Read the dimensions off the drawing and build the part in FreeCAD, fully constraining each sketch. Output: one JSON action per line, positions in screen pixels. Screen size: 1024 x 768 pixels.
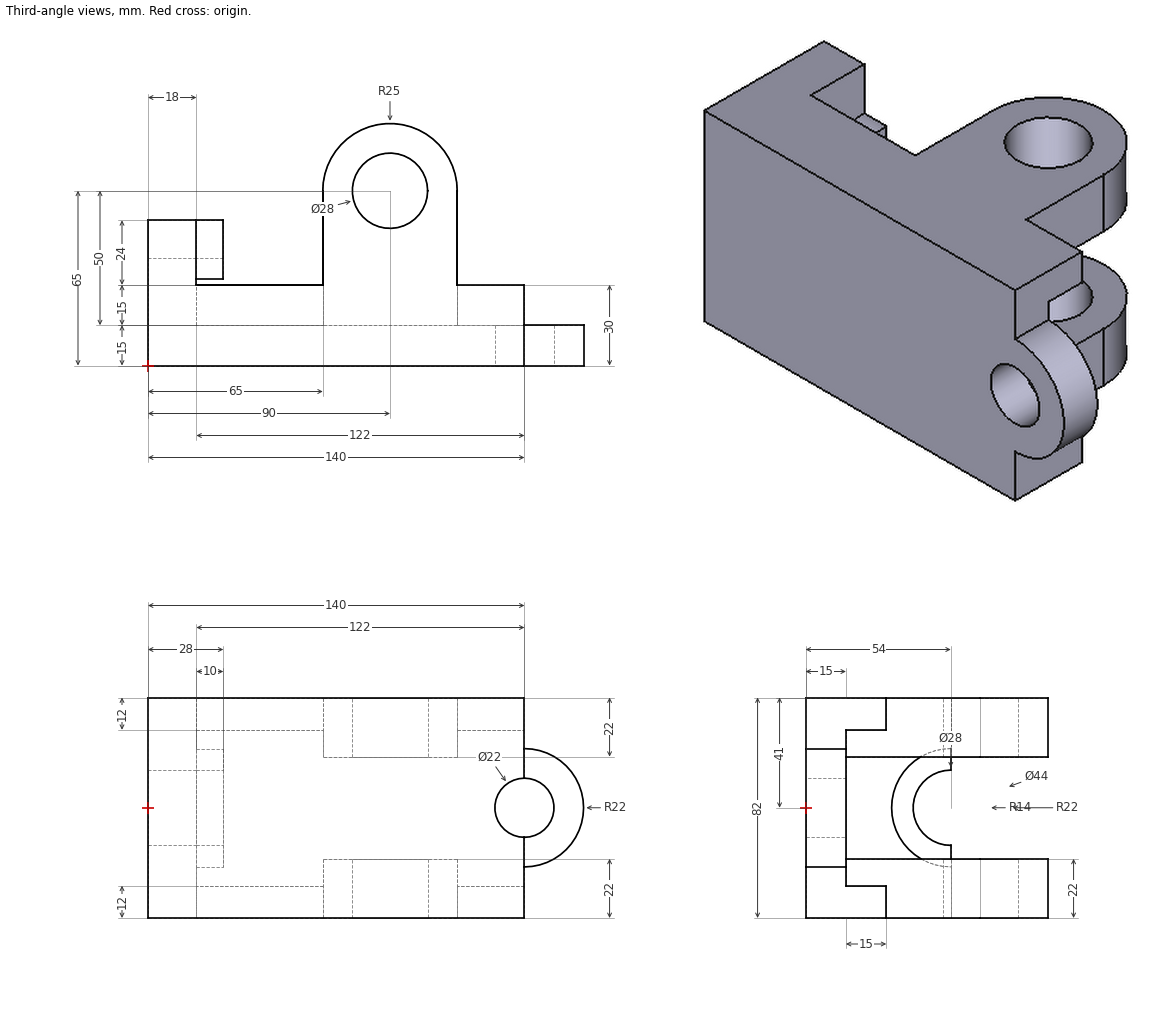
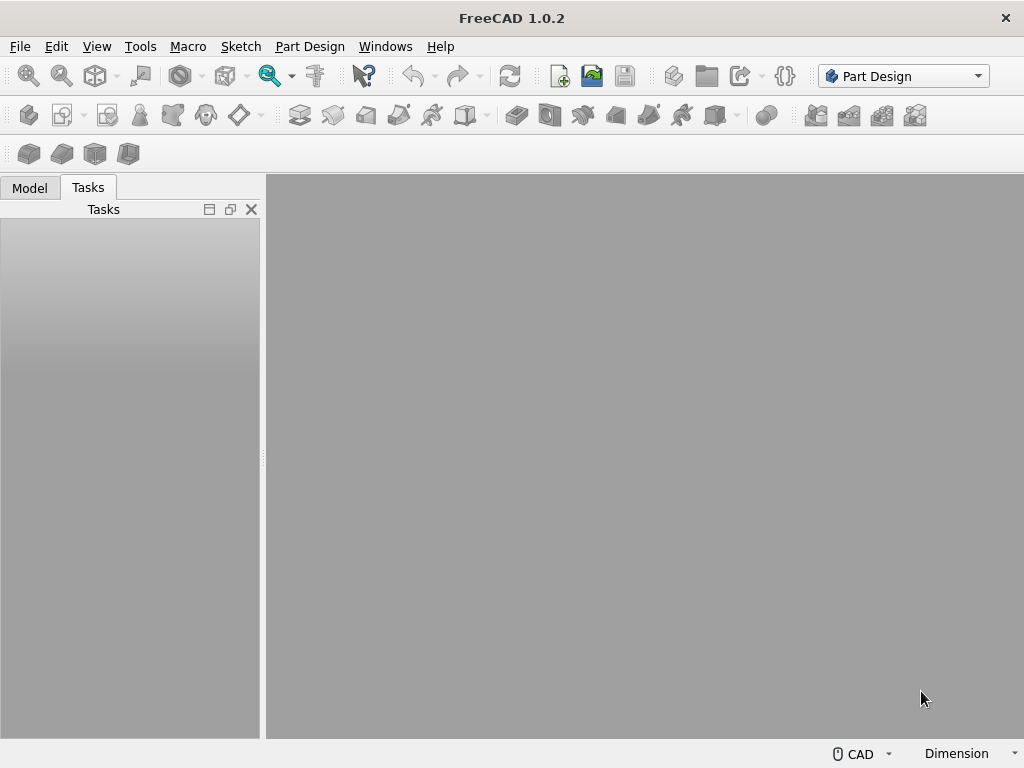
{"action": "key", "text": "ctrl+n"}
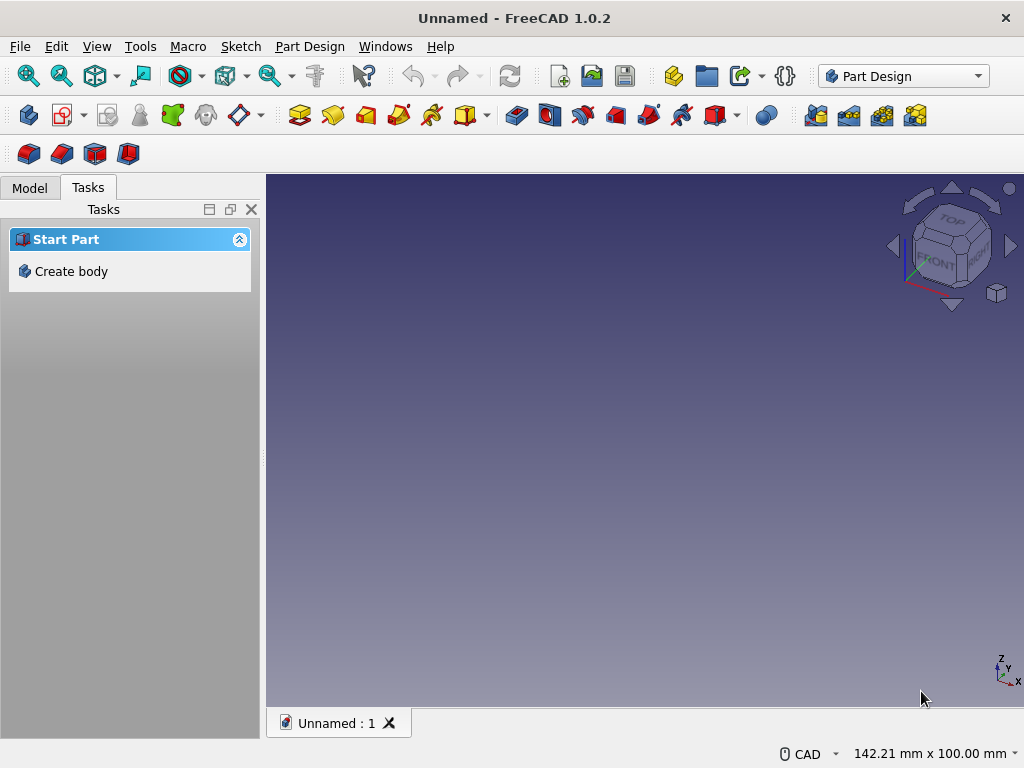
{"action": "left_click", "coordinate": [62, 116]}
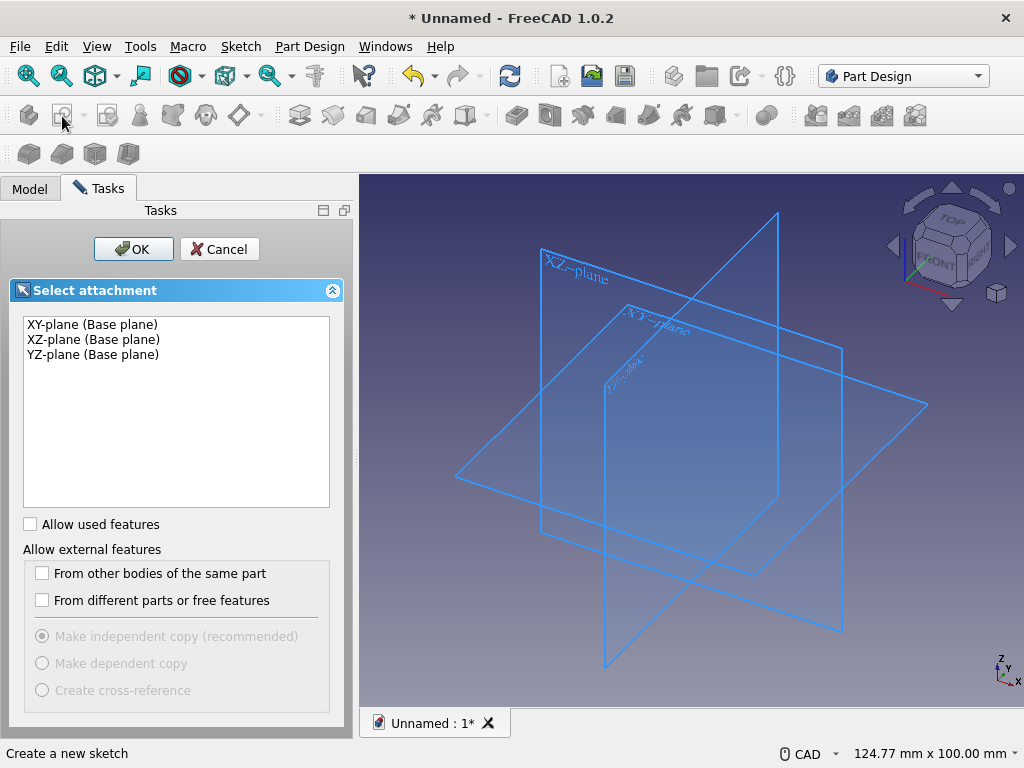
{"action": "left_click", "coordinate": [84, 324]}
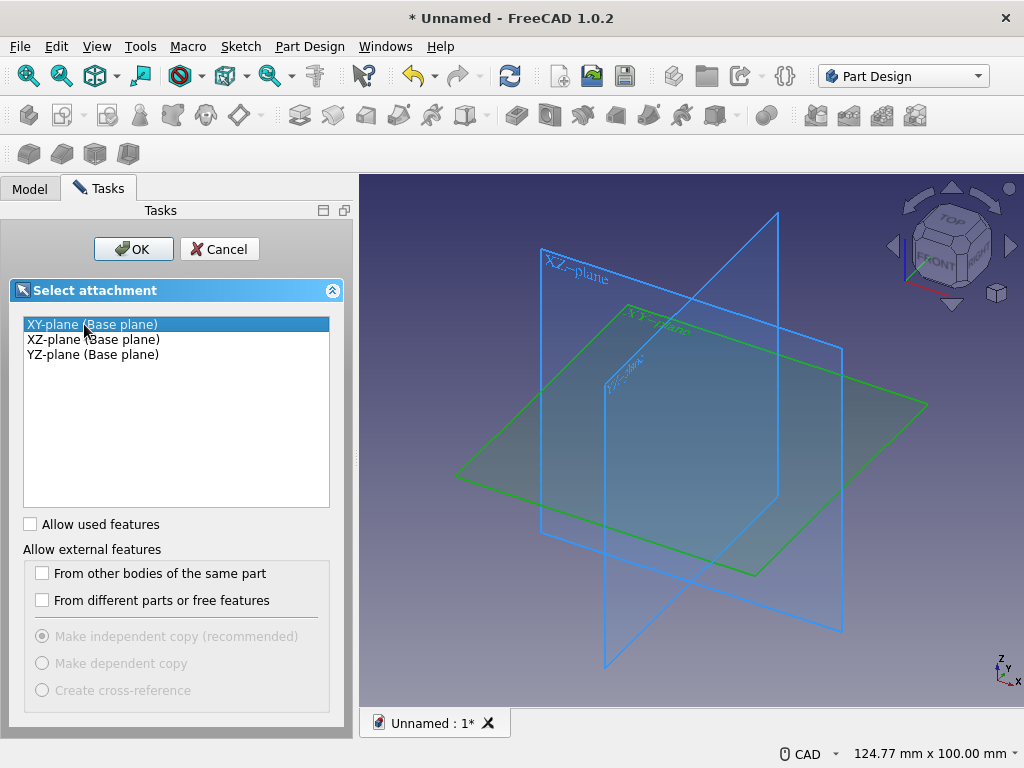
{"action": "left_click", "coordinate": [134, 249]}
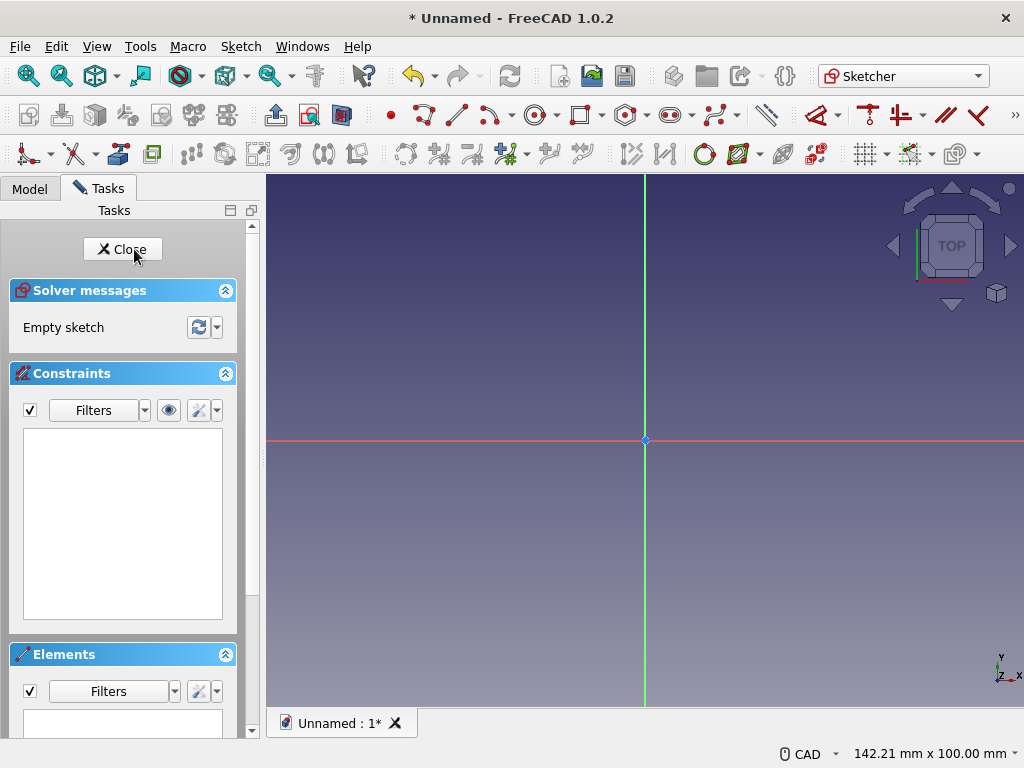
{"action": "scroll", "coordinate": [294, 558], "scroll_direction": "down", "scroll_amount": 4}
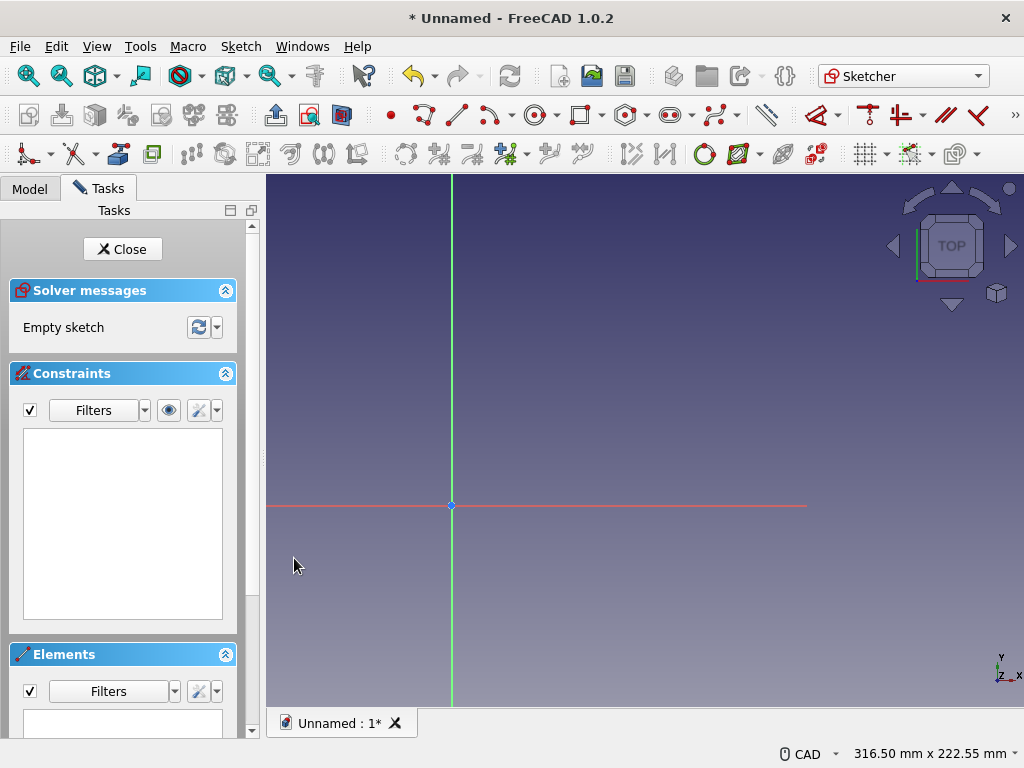
{"action": "left_click", "coordinate": [424, 116]}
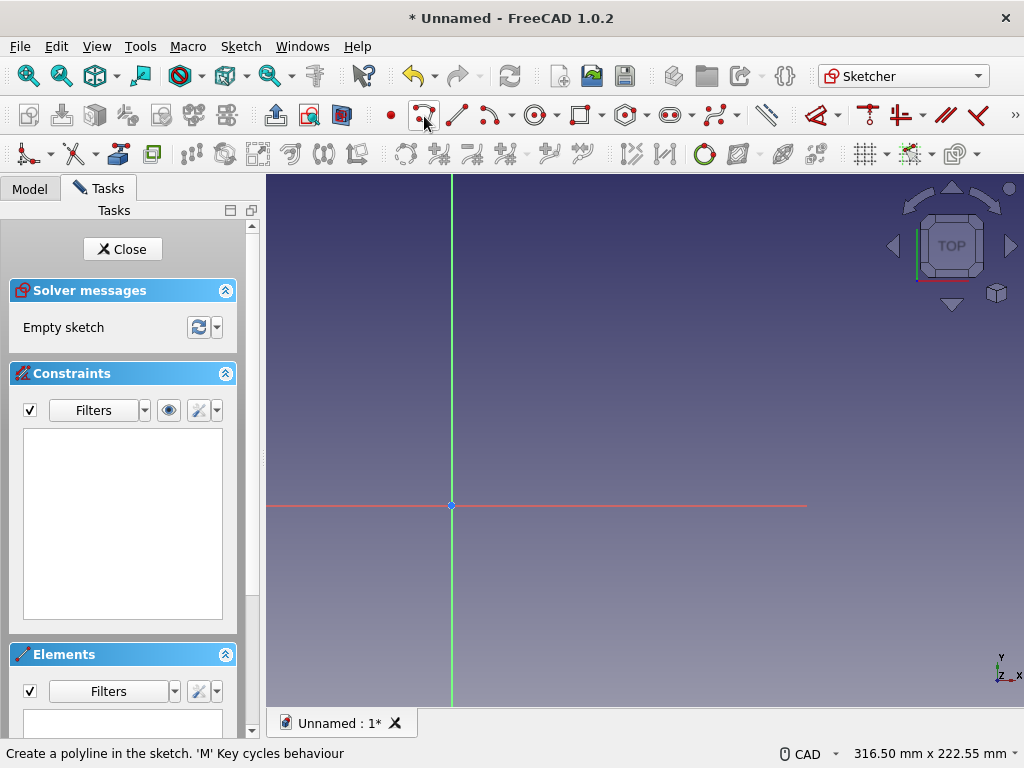
{"action": "left_click", "coordinate": [452, 506]}
{"action": "left_click", "coordinate": [787, 497]}
{"action": "left_click", "coordinate": [787, 434]}
{"action": "left_click", "coordinate": [495, 434]}
{"action": "left_click", "coordinate": [495, 376]}
{"action": "left_click", "coordinate": [461, 376]}
{"action": "left_click", "coordinate": [452, 506]}
{"action": "key", "text": "Escape"}
{"action": "key", "text": "Escape"}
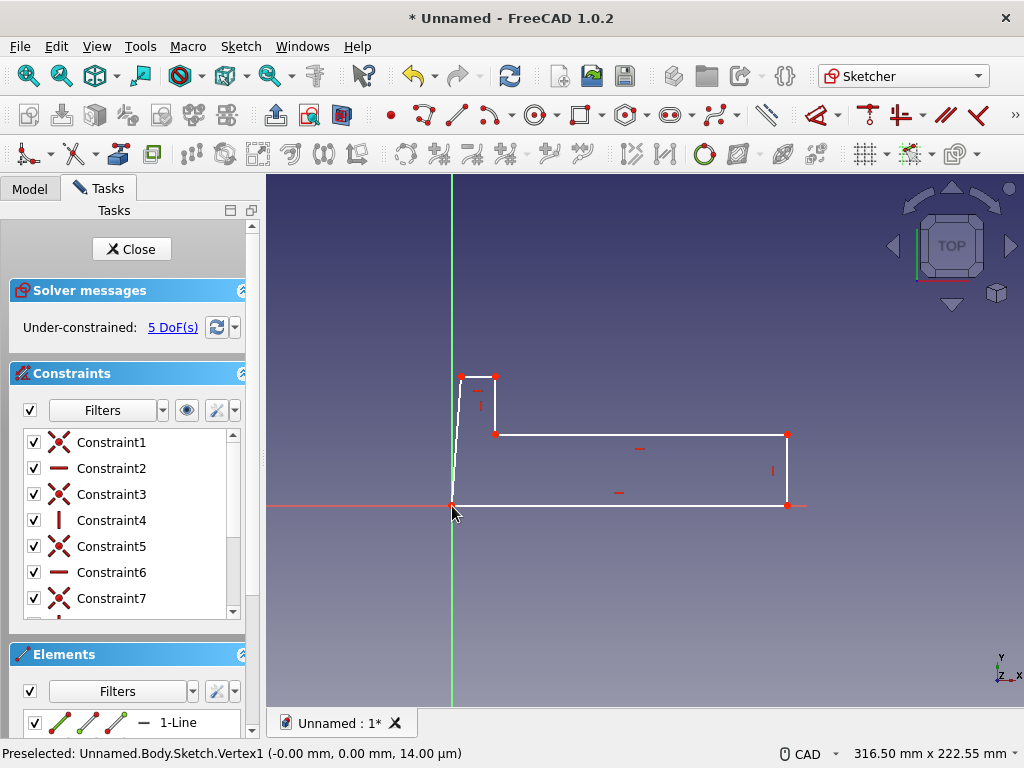
{"action": "left_click", "coordinate": [455, 467]}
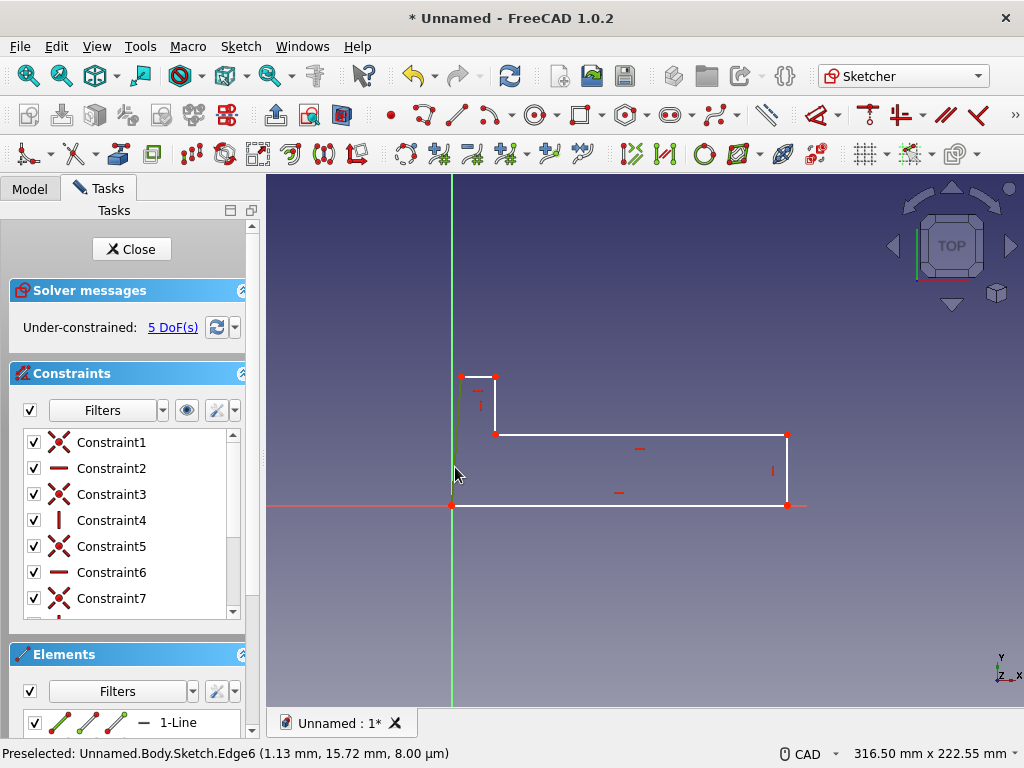
{"action": "key", "text": "v"}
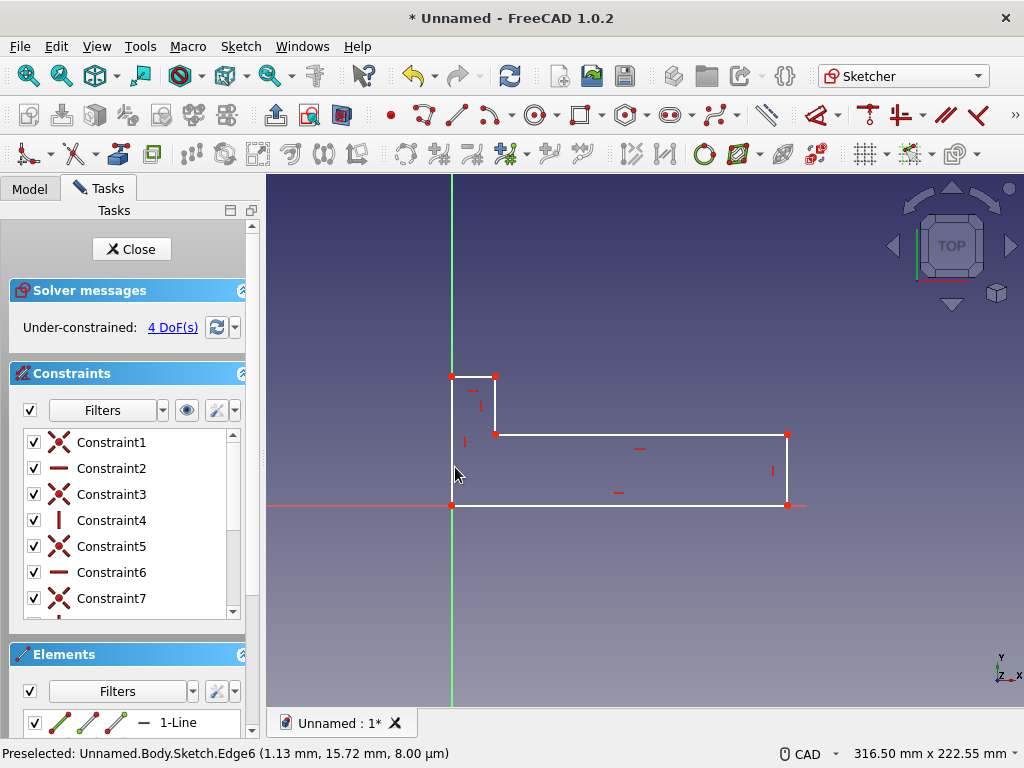
{"action": "key", "text": "d"}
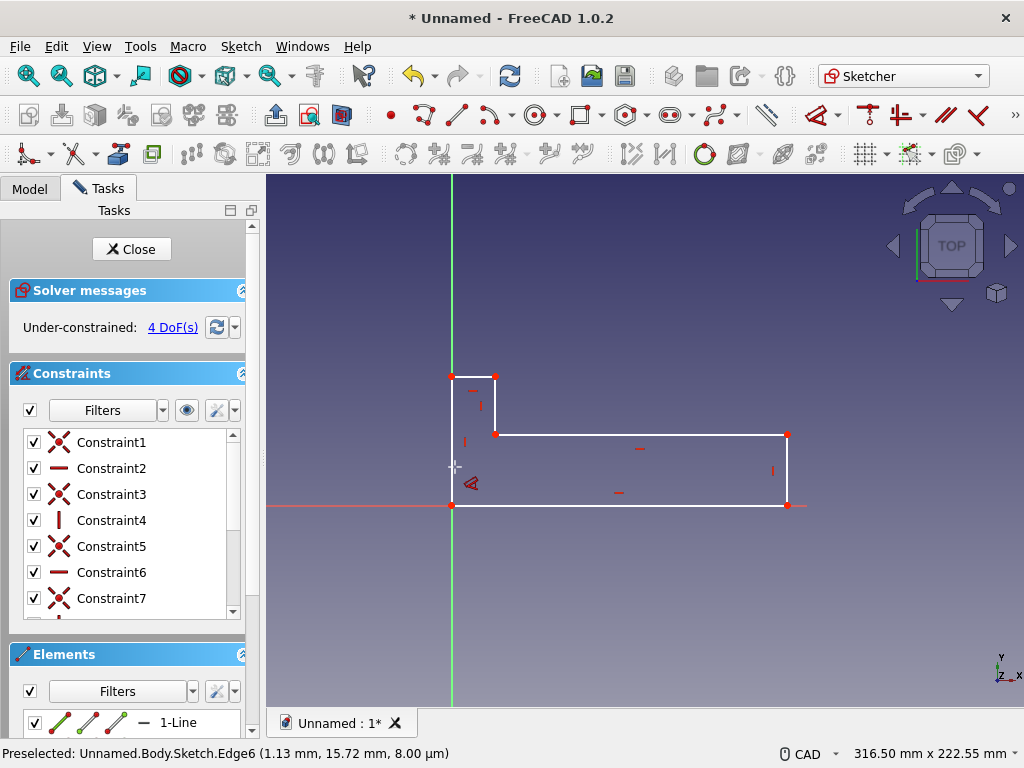
{"action": "left_click", "coordinate": [787, 484]}
{"action": "left_click", "coordinate": [821, 470]}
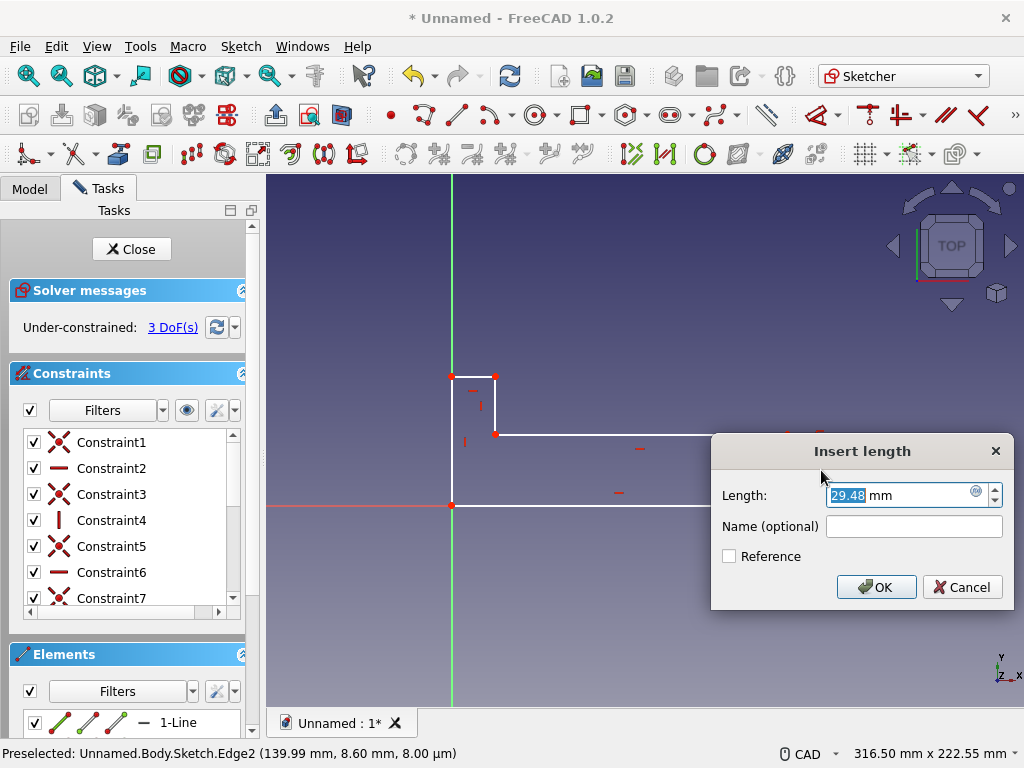
{"action": "type", "text": "30"}
{"action": "key", "text": "Return"}